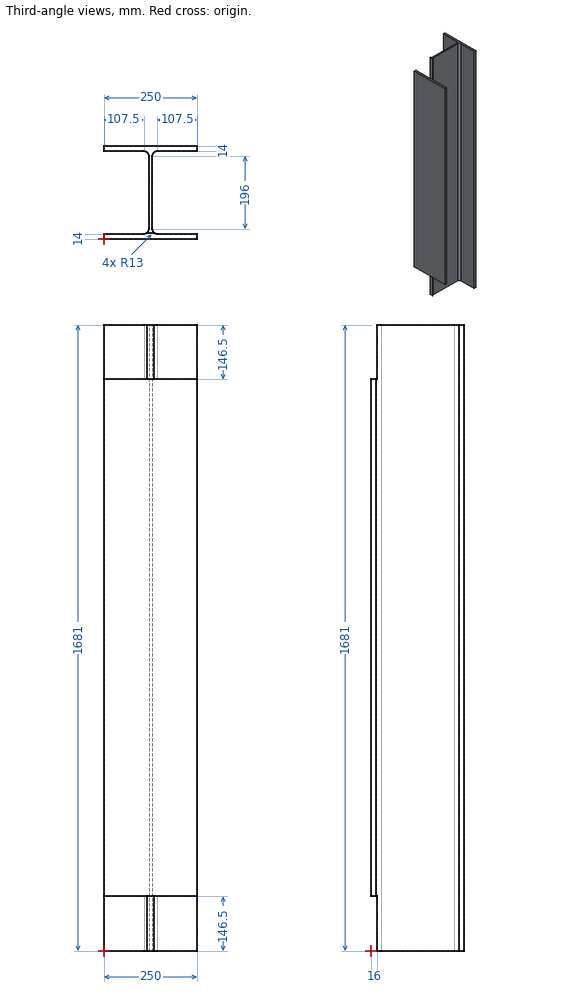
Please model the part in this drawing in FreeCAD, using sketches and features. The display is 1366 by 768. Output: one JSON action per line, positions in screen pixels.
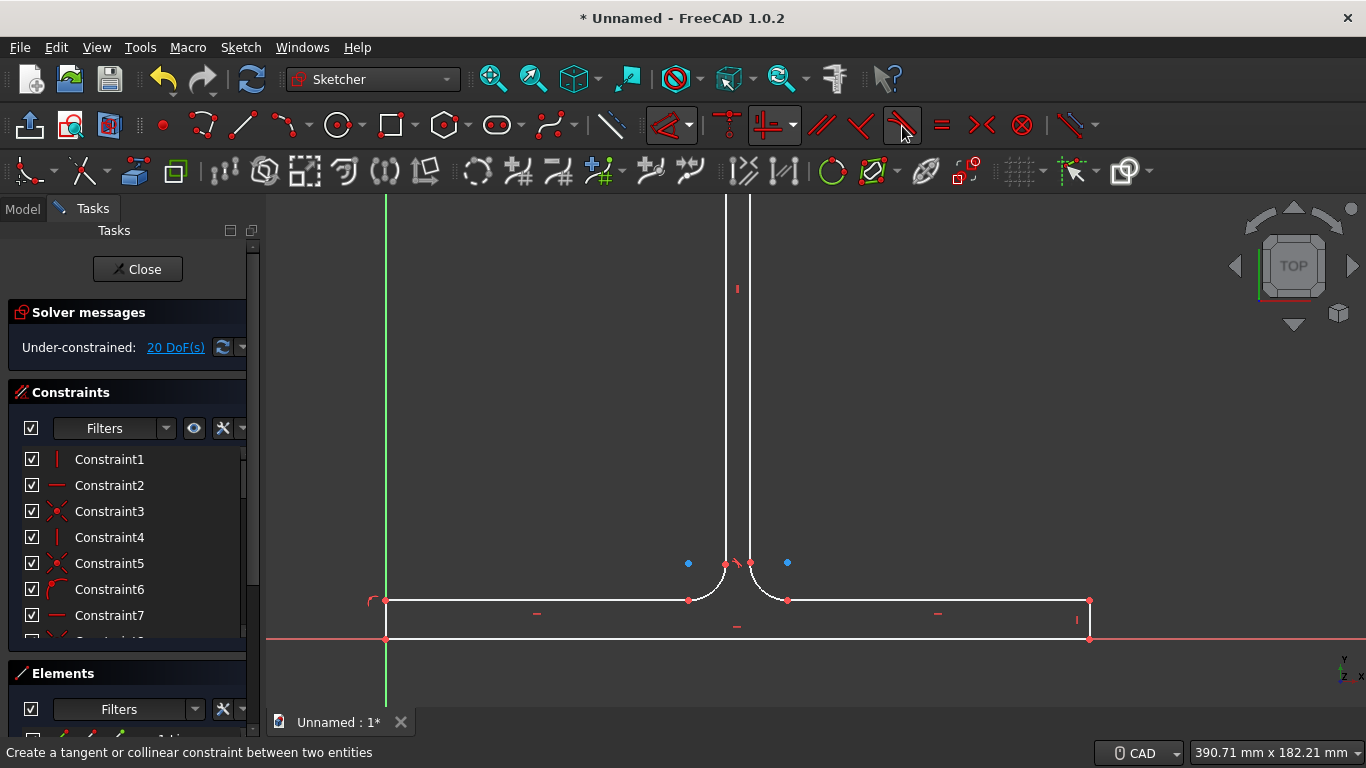
{"action": "scroll", "coordinate": [755, 584], "scroll_direction": "down", "scroll_amount": 4}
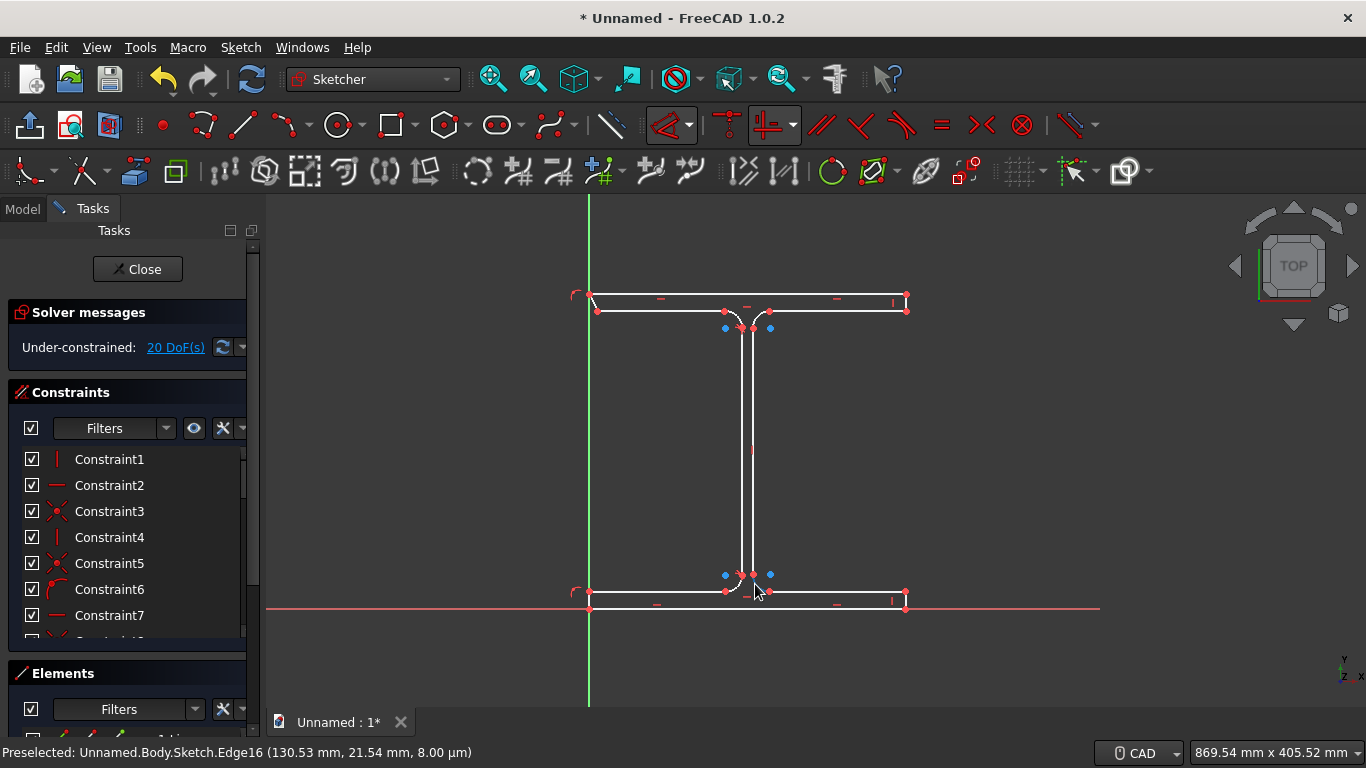
{"action": "left_click", "coordinate": [811, 311]}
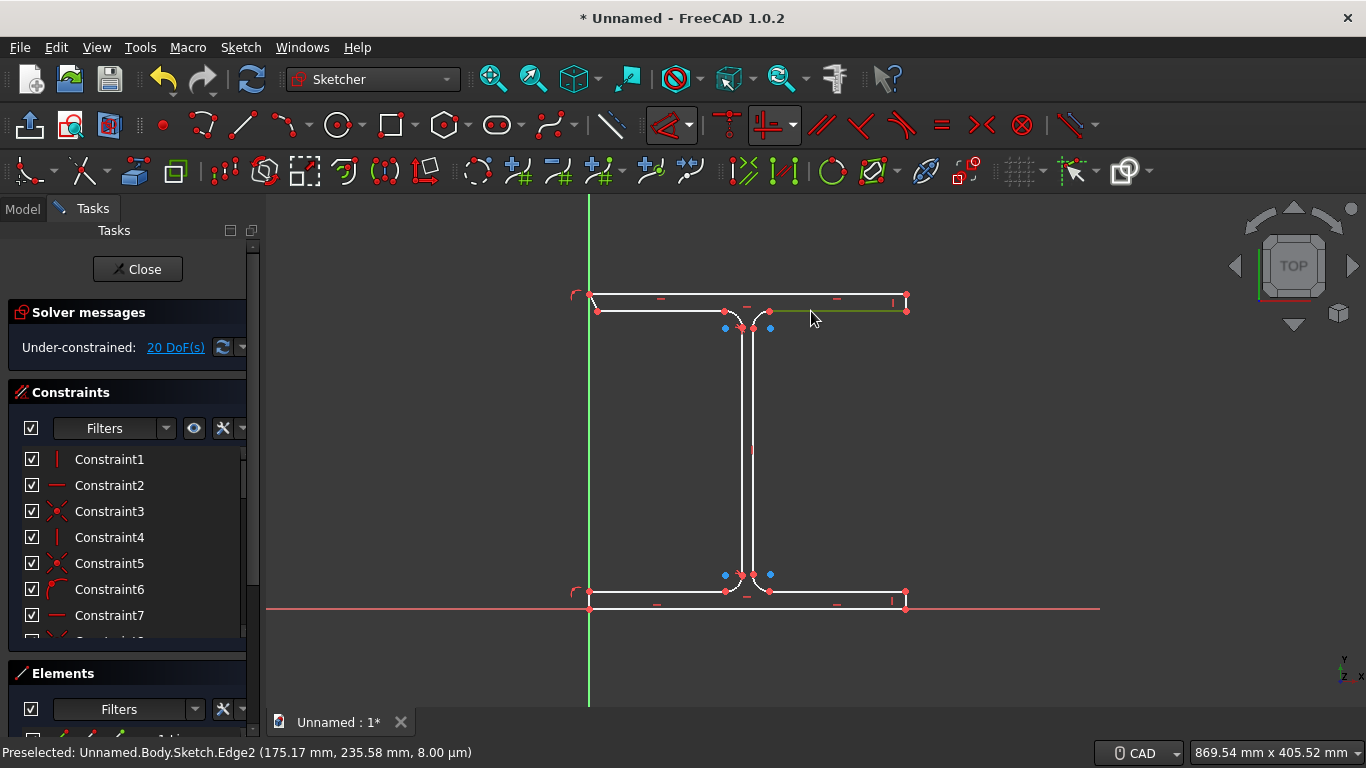
{"action": "left_click", "coordinate": [758, 316]}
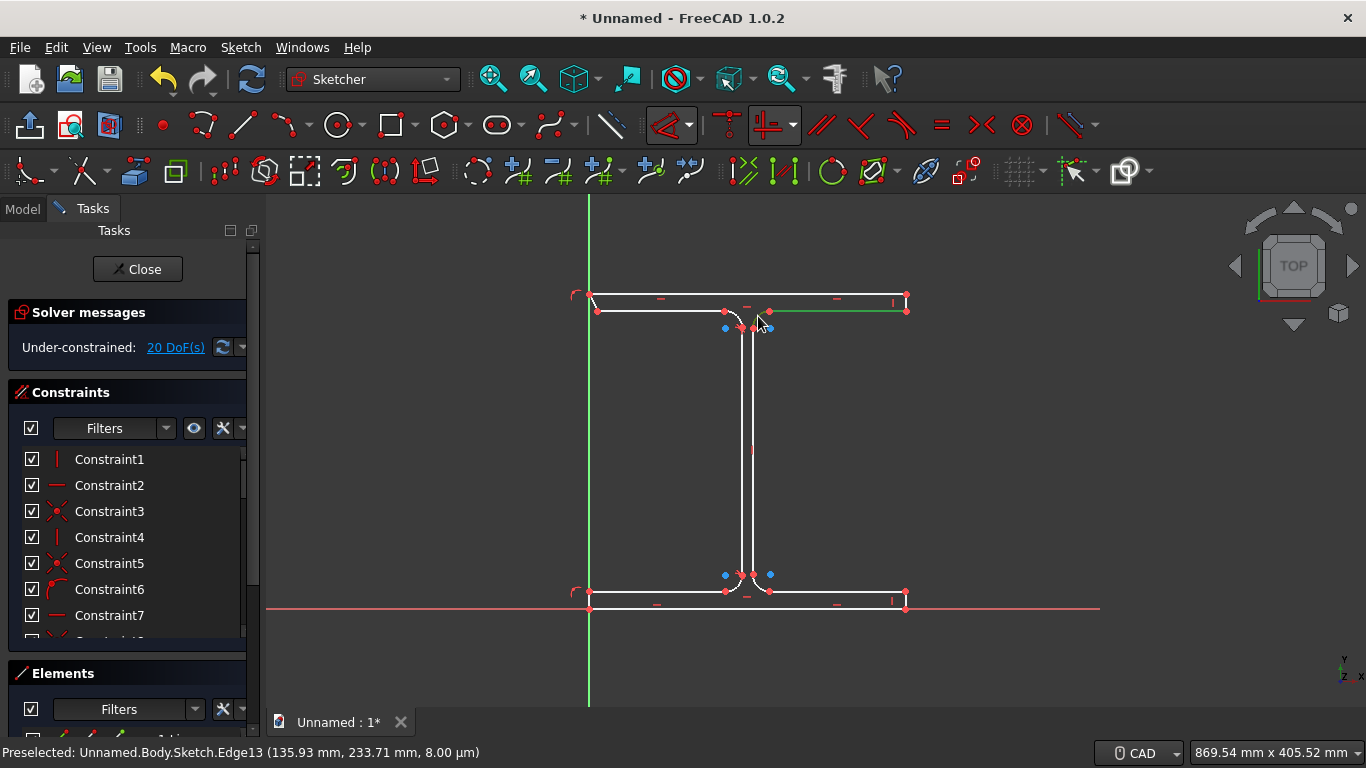
{"action": "left_click", "coordinate": [902, 126]}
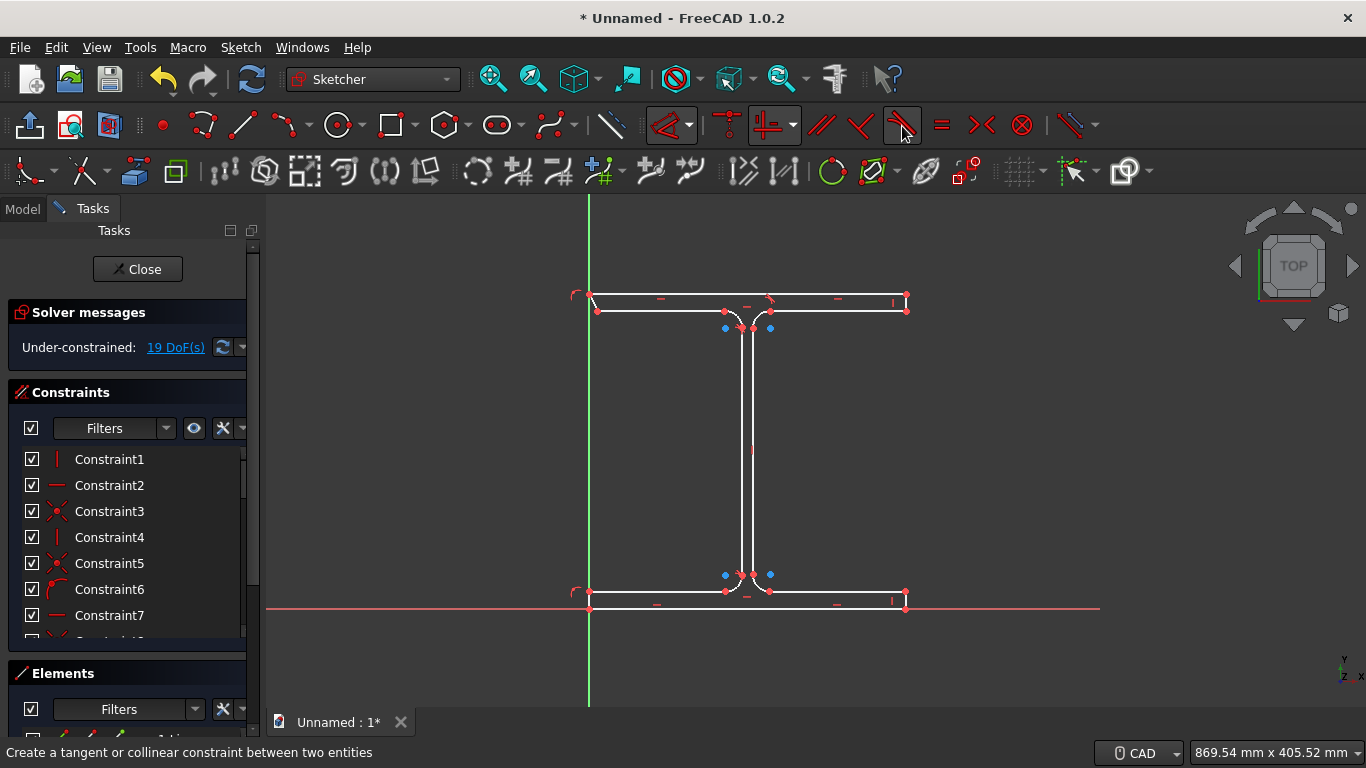
{"action": "left_click", "coordinate": [636, 311]}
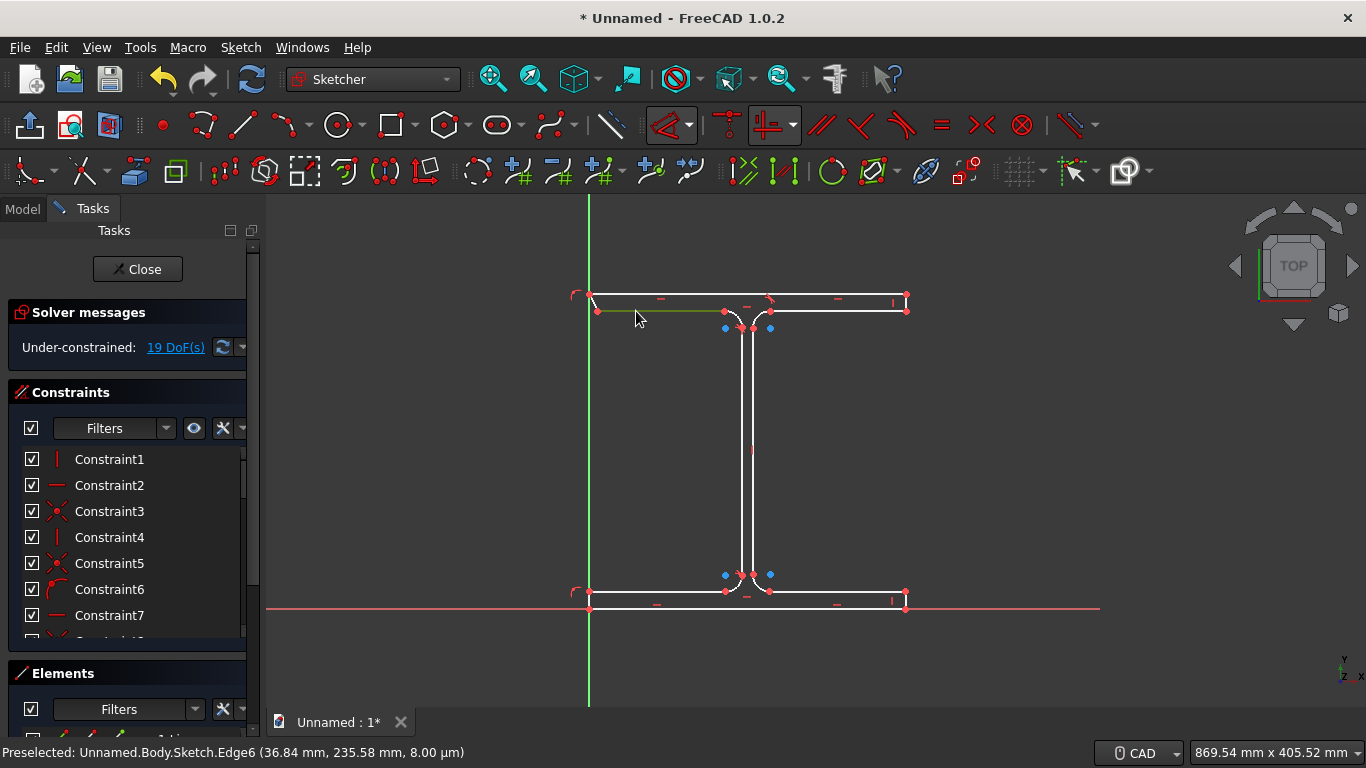
{"action": "left_click", "coordinate": [737, 316]}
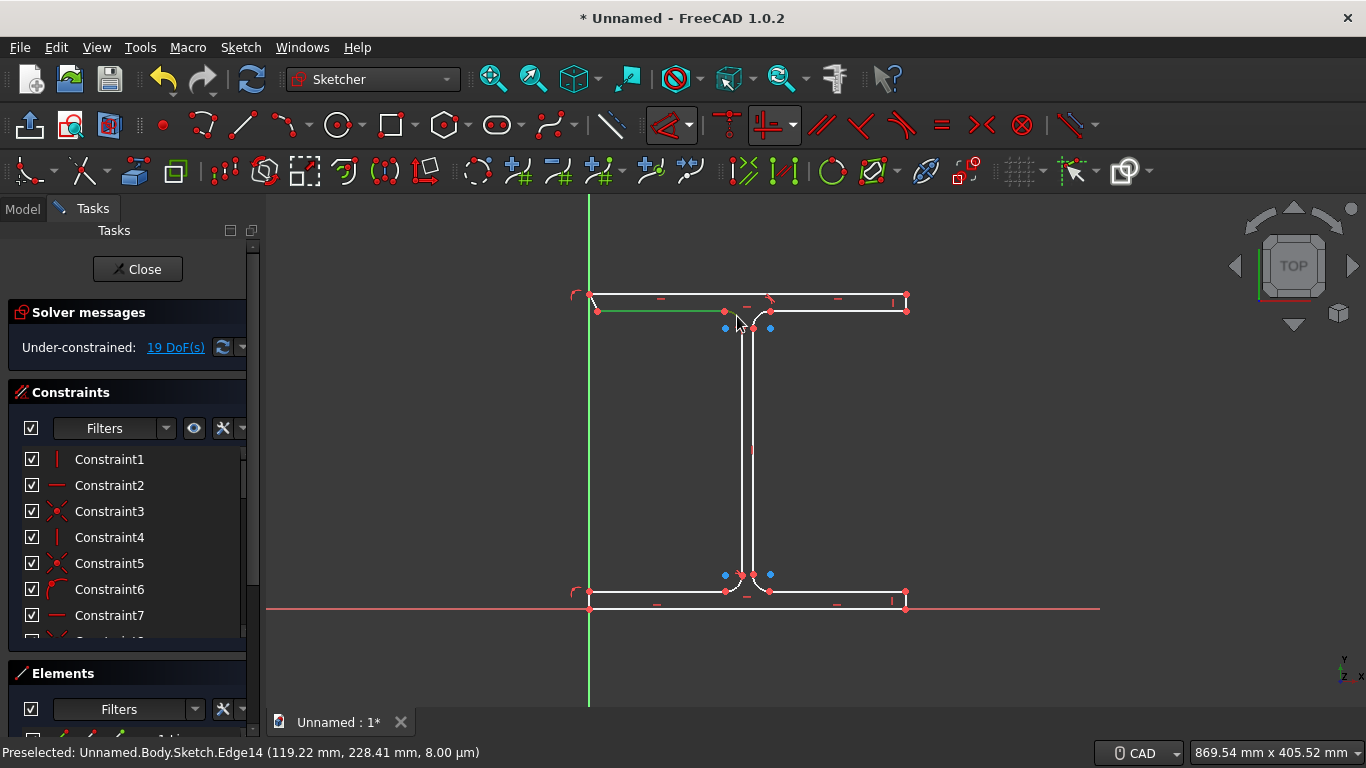
{"action": "left_click", "coordinate": [902, 126]}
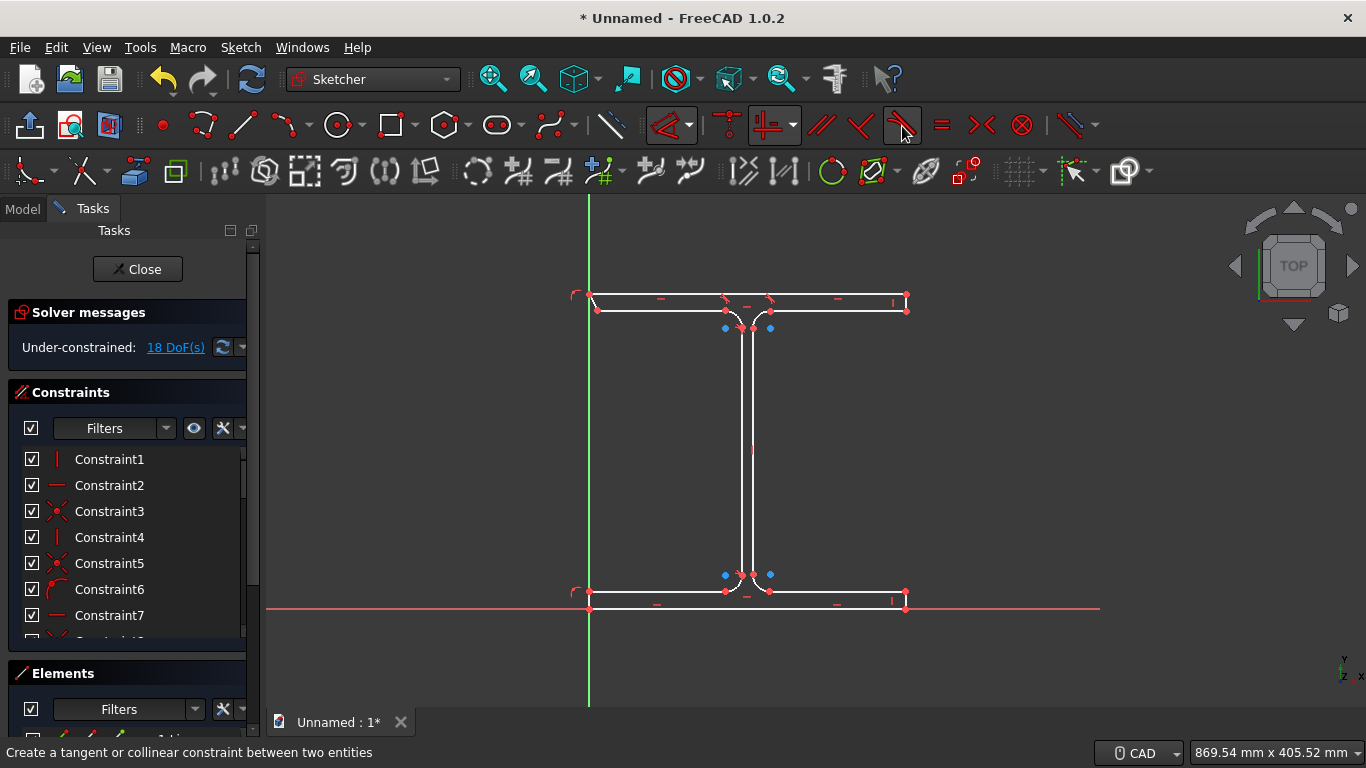
{"action": "scroll", "coordinate": [742, 402], "scroll_direction": "up", "scroll_amount": 2}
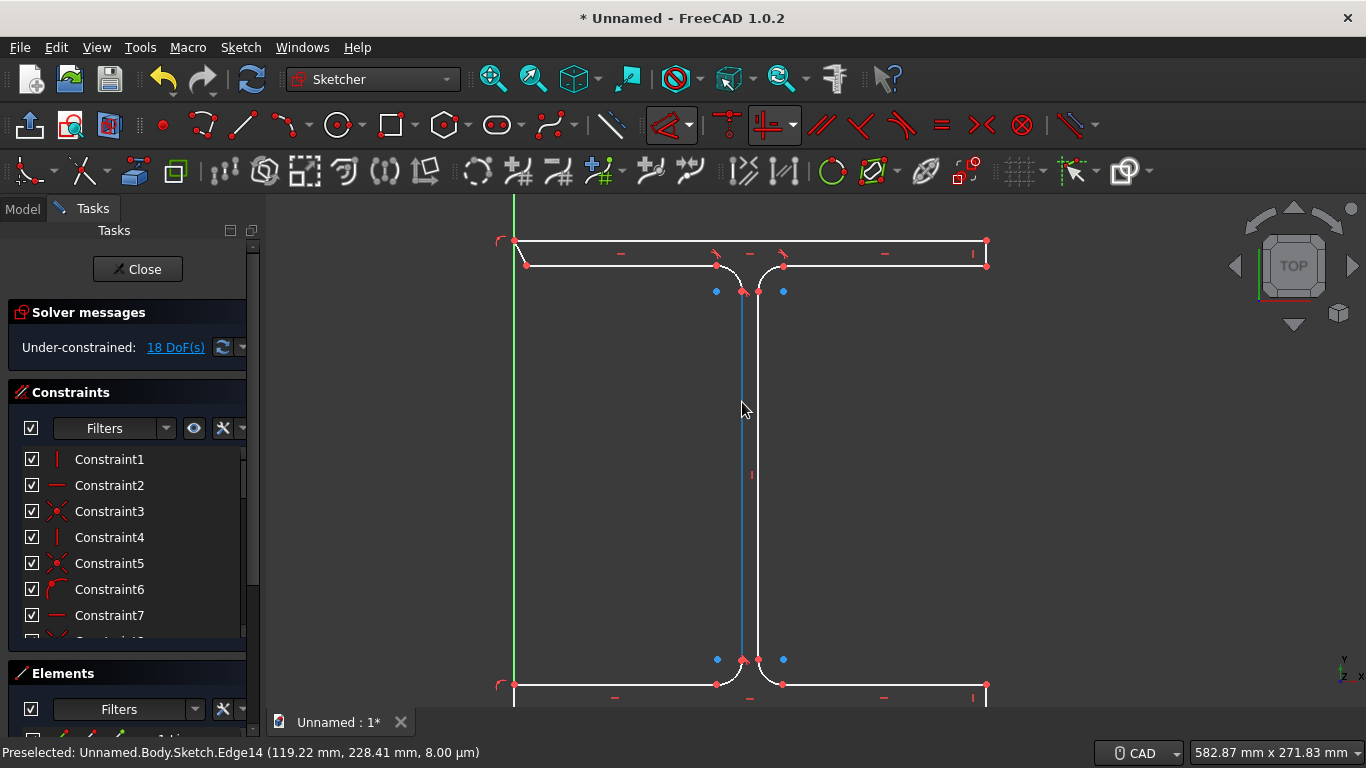
{"action": "left_click", "coordinate": [742, 402]}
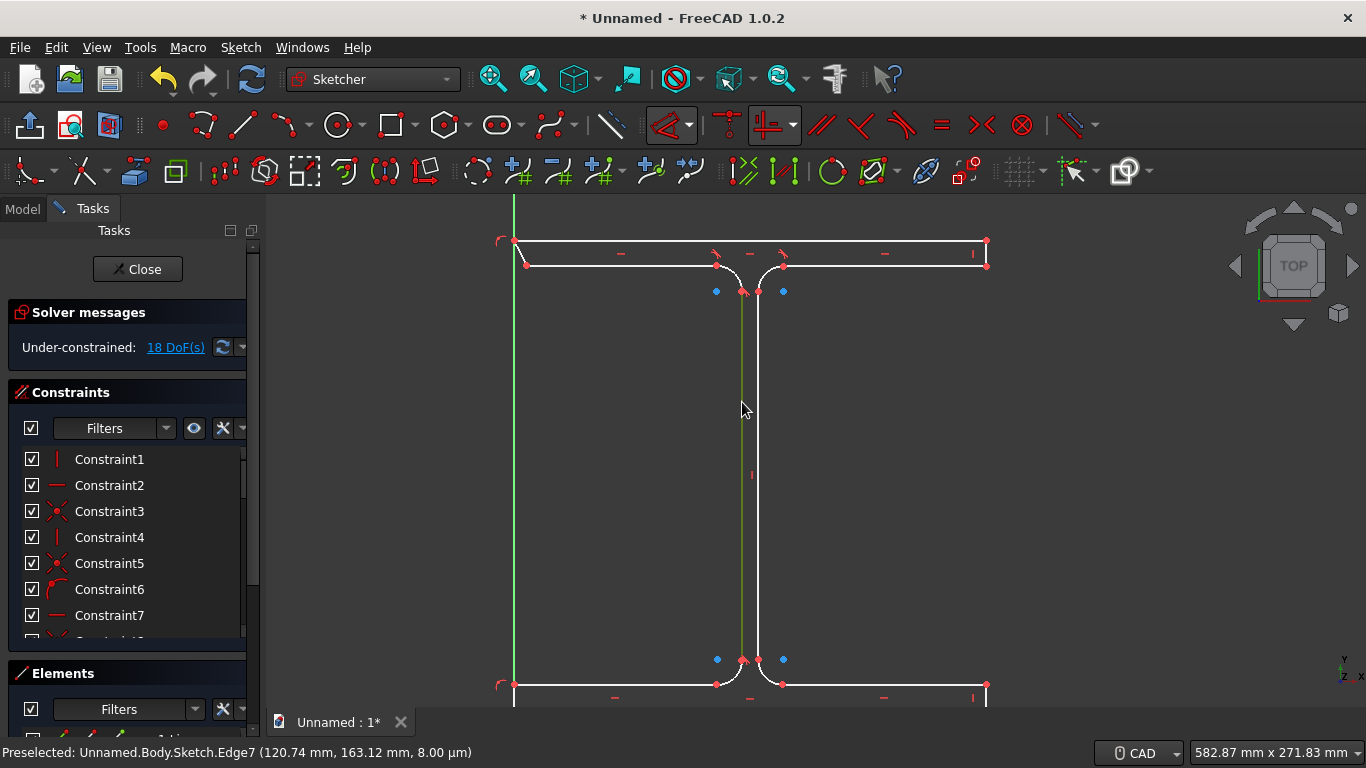
{"action": "left_click", "coordinate": [739, 280]}